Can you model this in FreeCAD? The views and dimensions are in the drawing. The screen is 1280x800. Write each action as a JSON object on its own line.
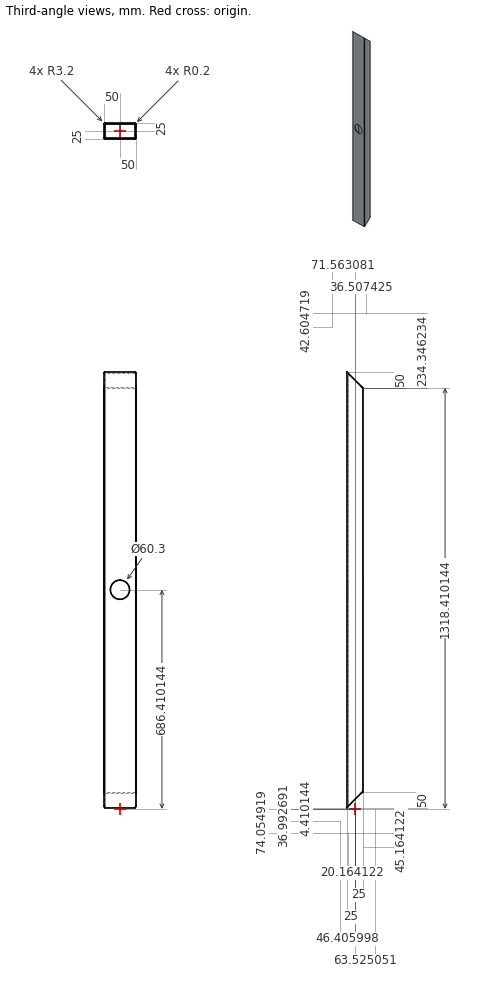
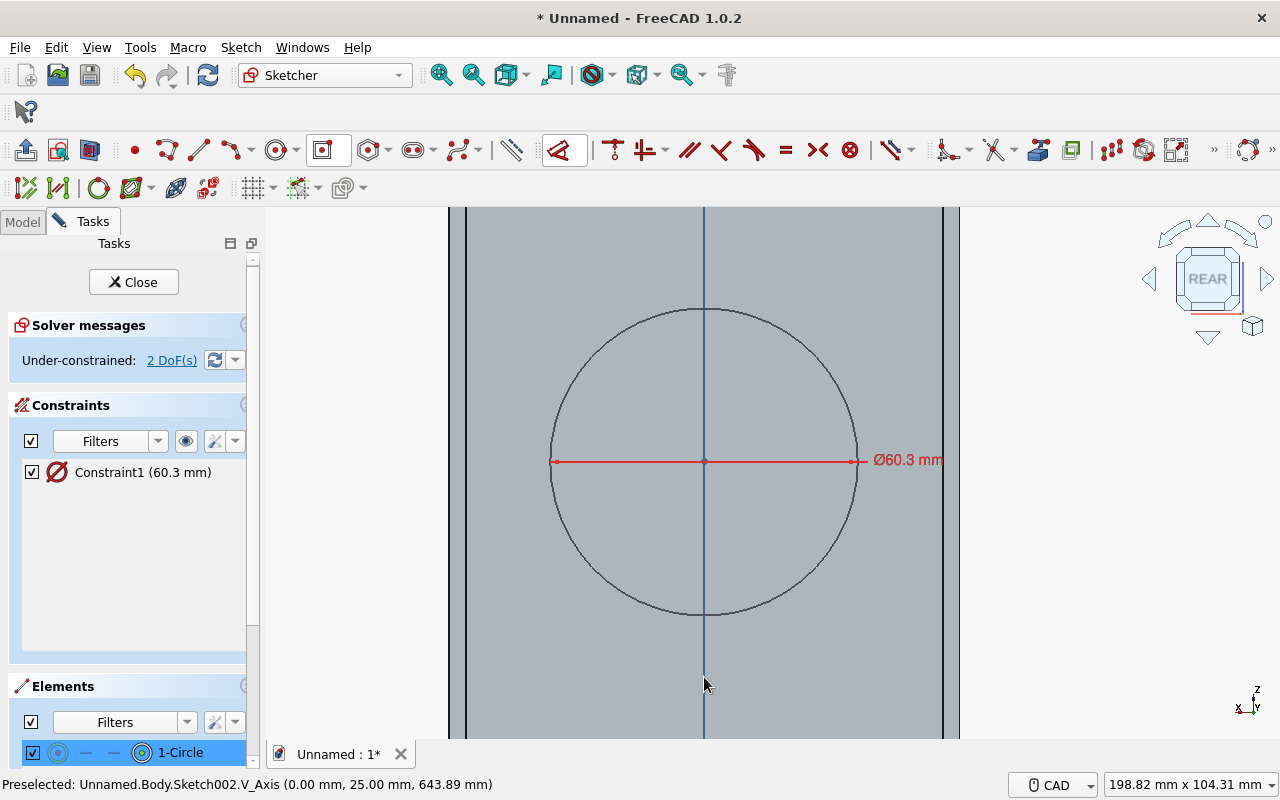
{"action": "left_click", "coordinate": [614, 150]}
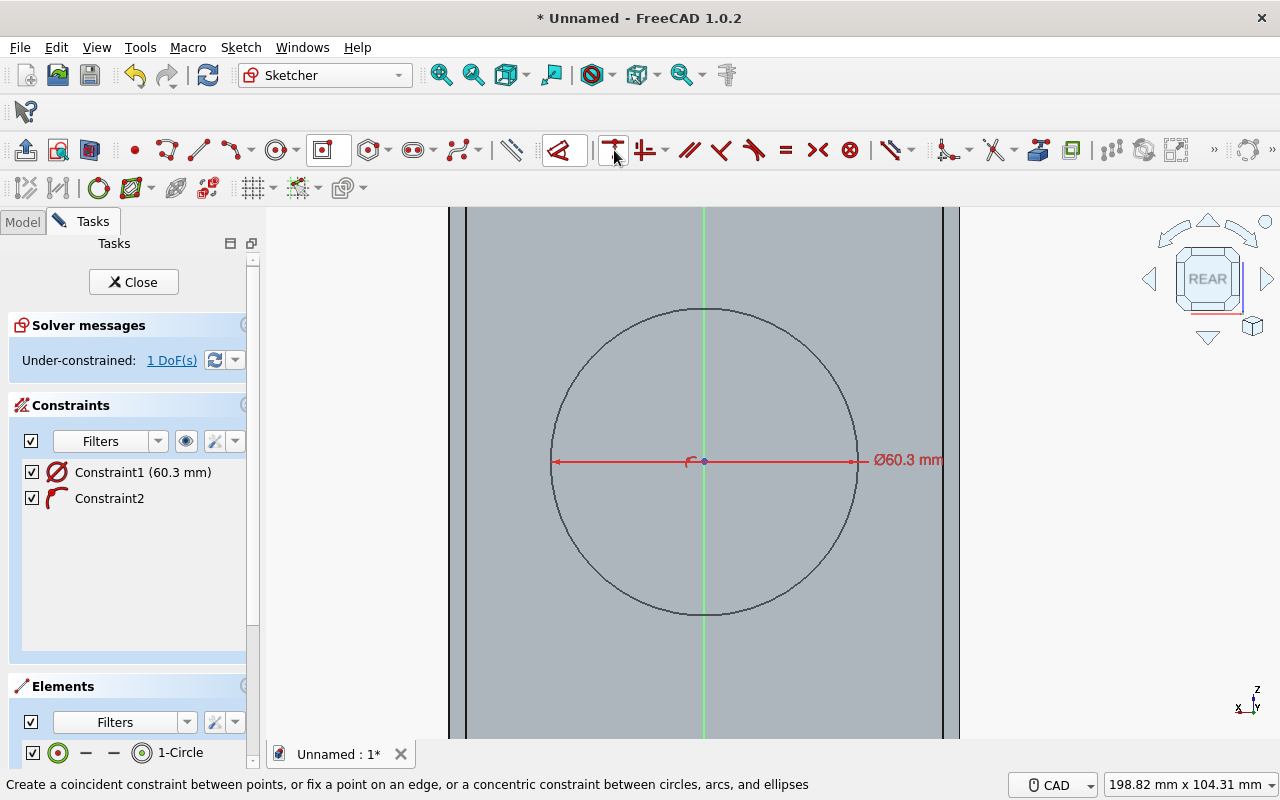
{"action": "left_click", "coordinate": [704, 462]}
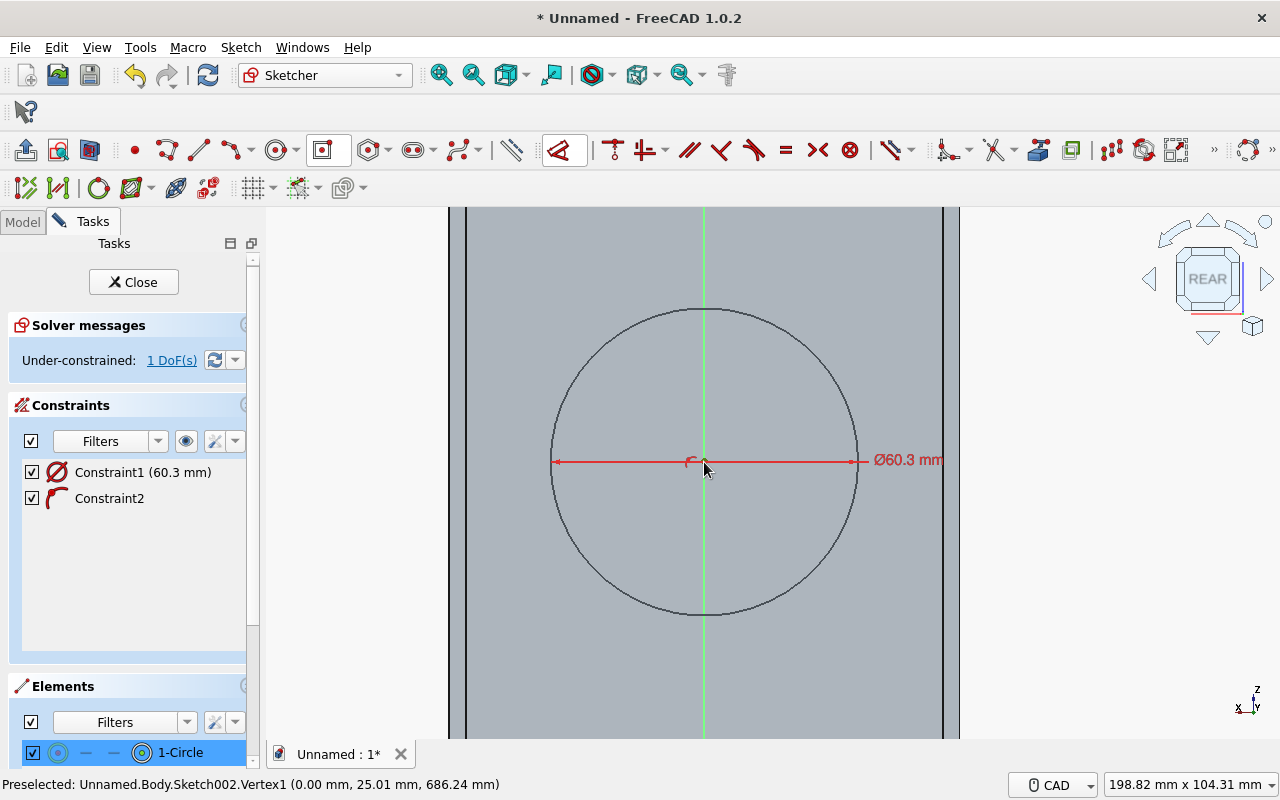
{"action": "left_click", "coordinate": [582, 150]}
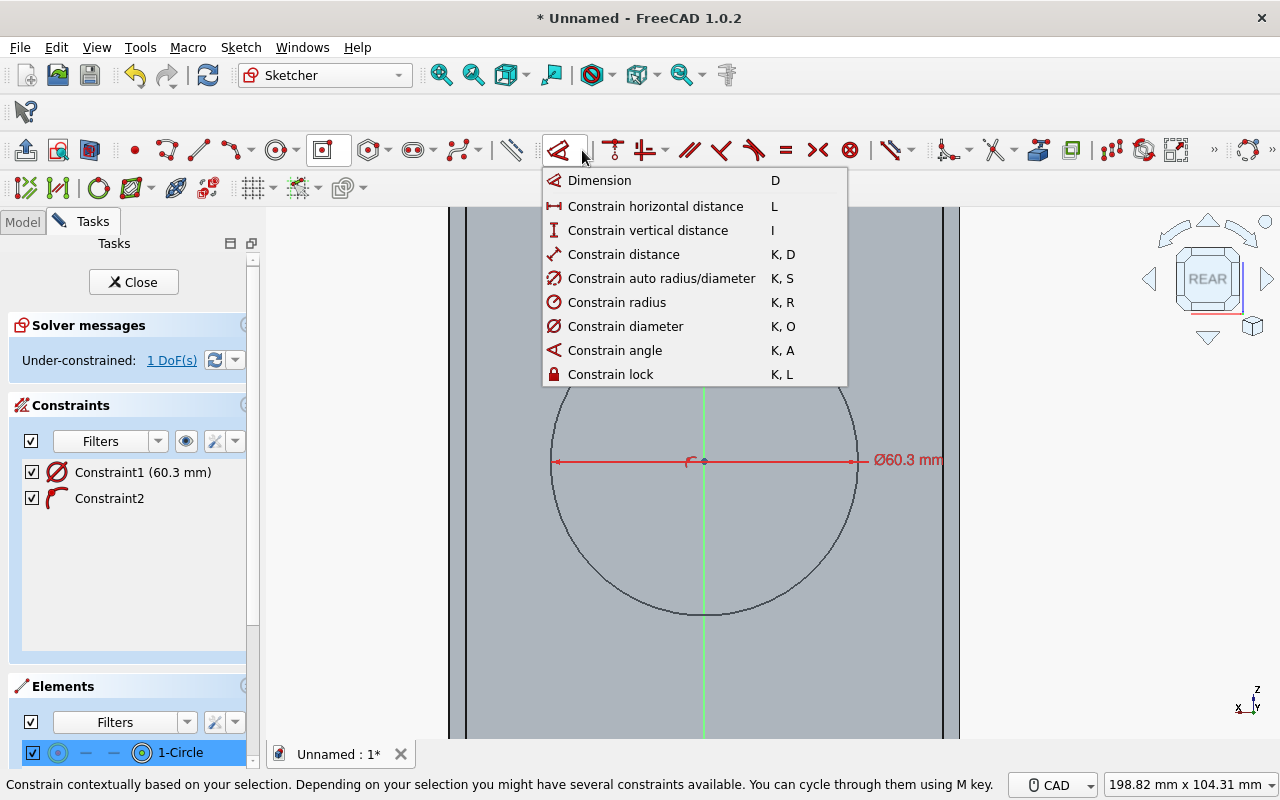
{"action": "left_click", "coordinate": [695, 230]}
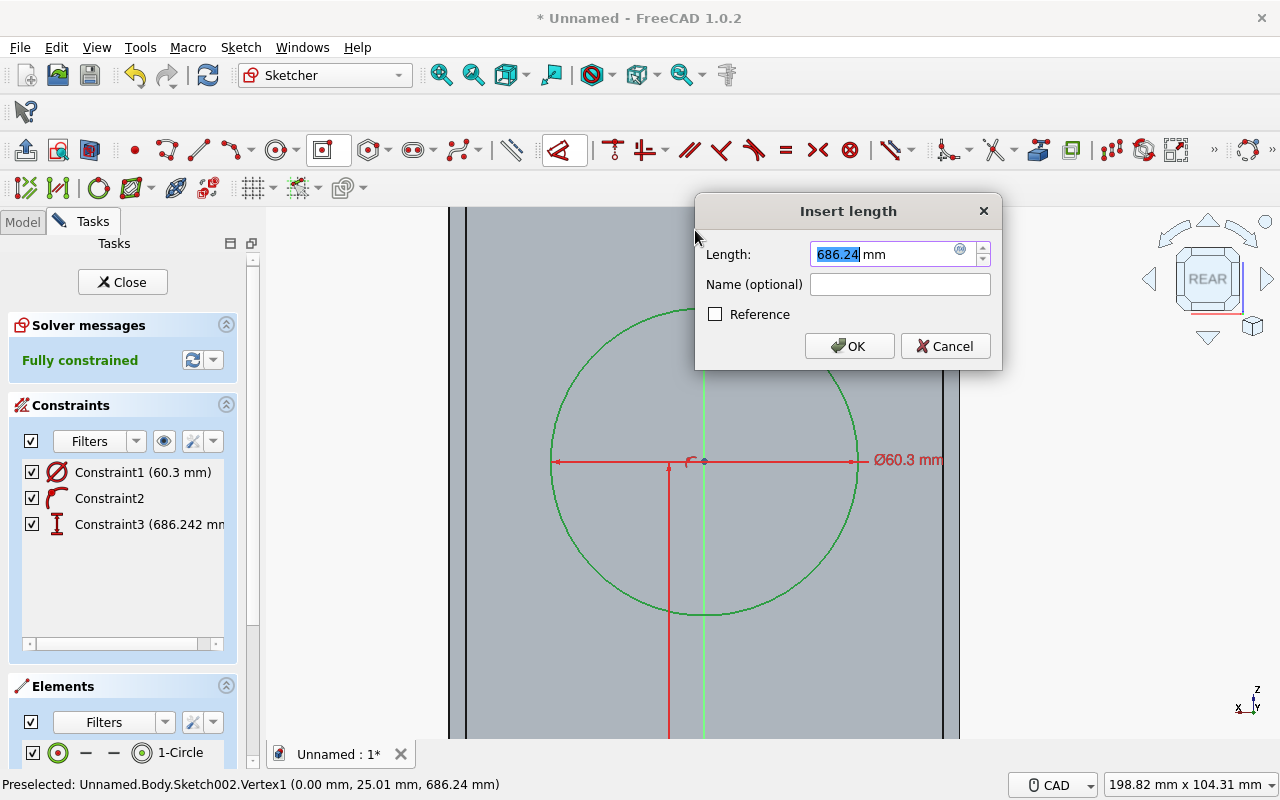
{"action": "type", "text": "686.410144"}
{"action": "key", "text": "Return"}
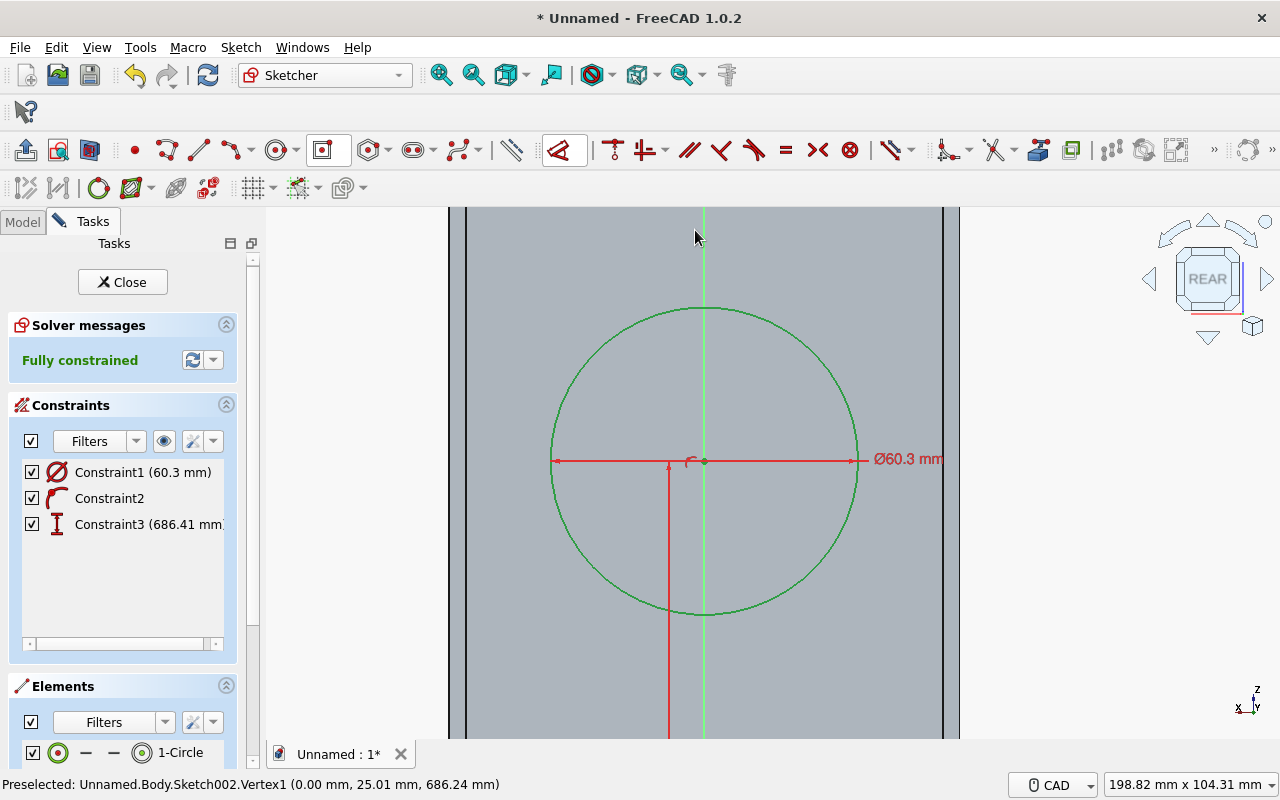
{"action": "left_click", "coordinate": [123, 282]}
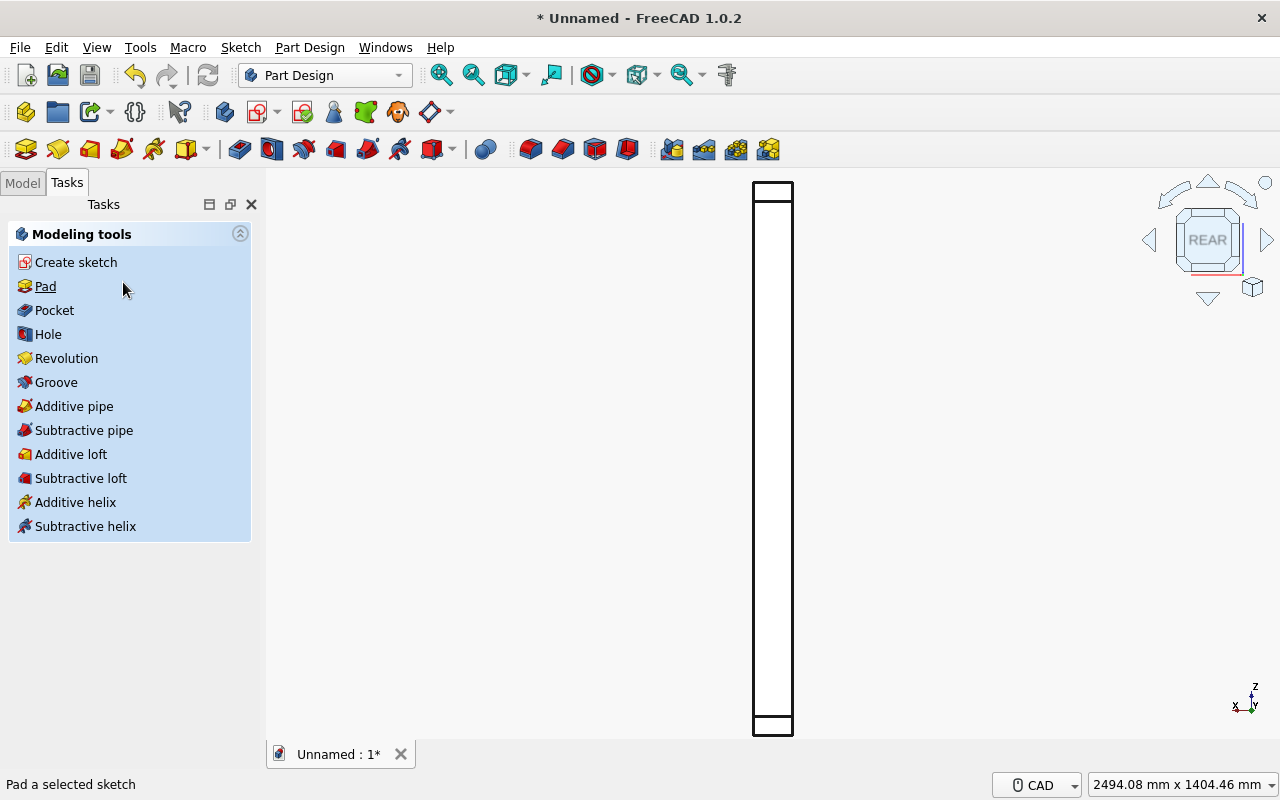
{"action": "left_click", "coordinate": [240, 150]}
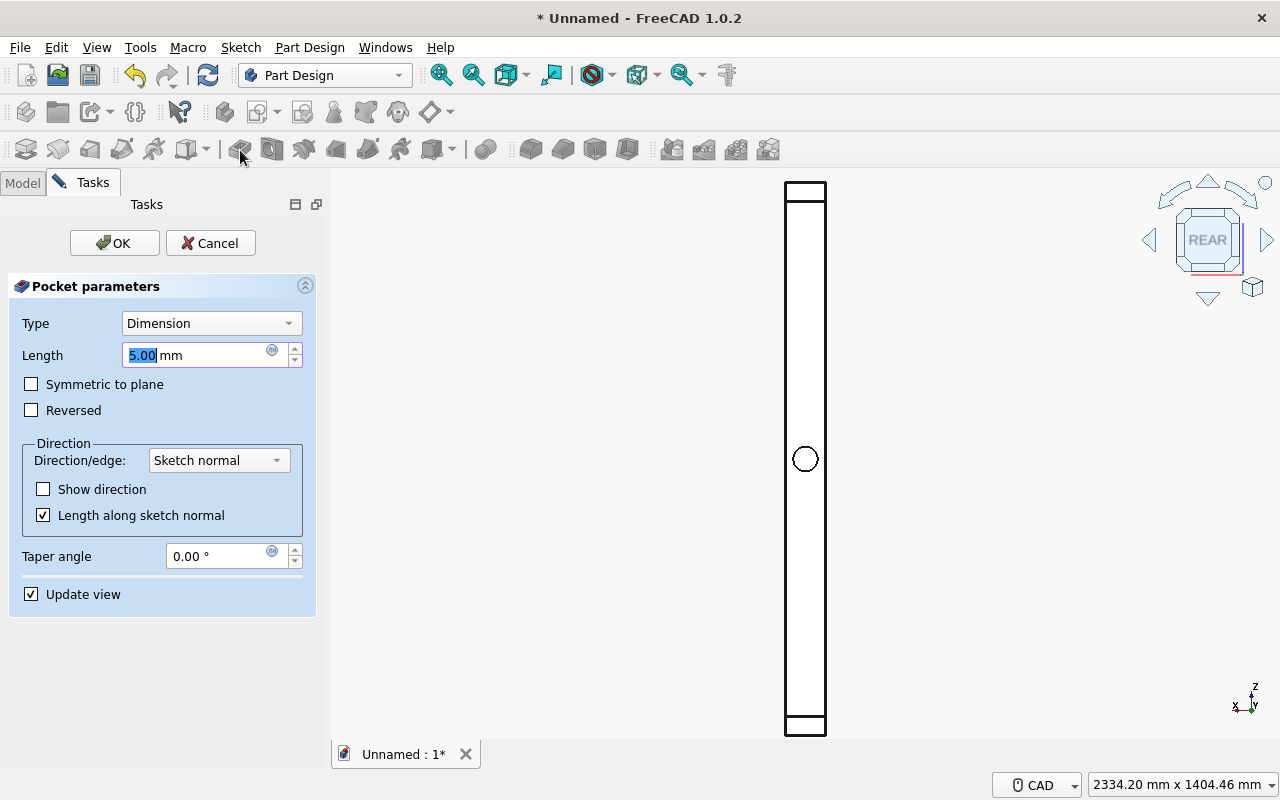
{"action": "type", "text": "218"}
{"action": "key", "text": "Tab"}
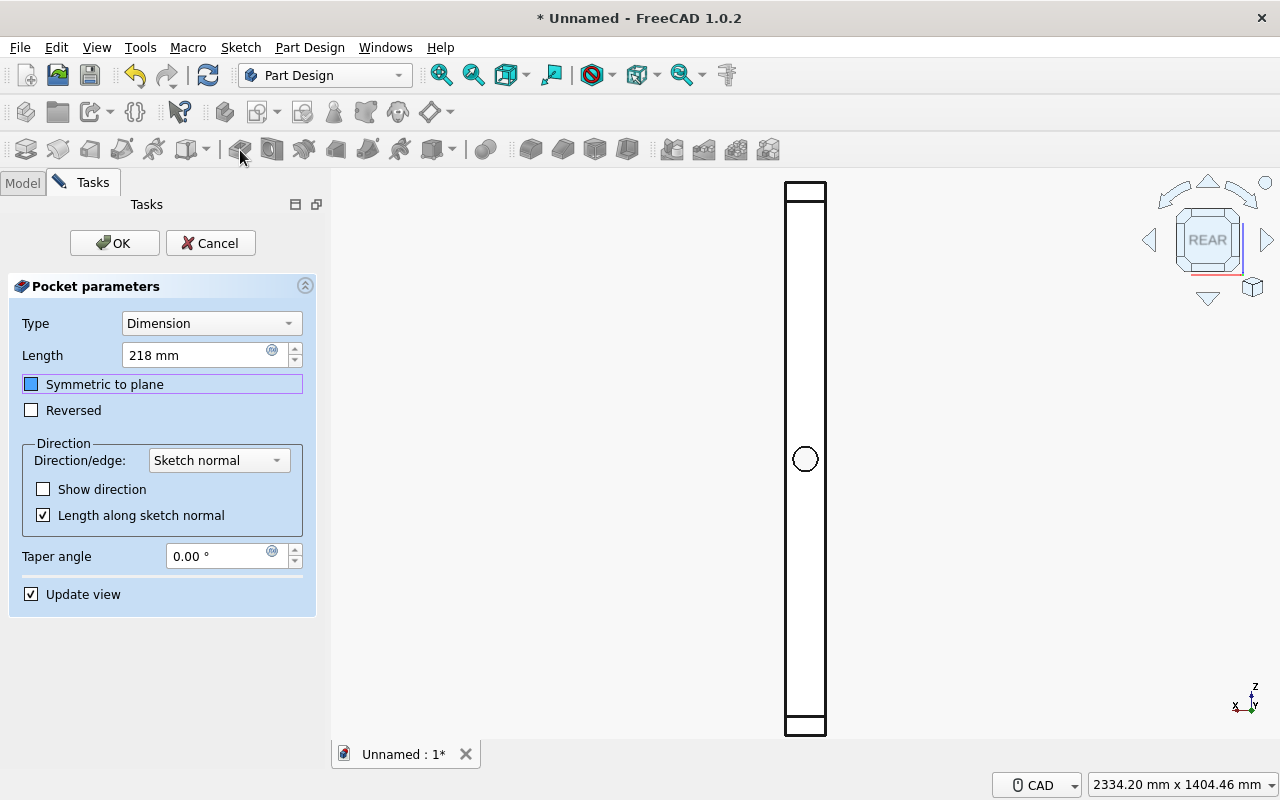
{"action": "left_click", "coordinate": [115, 243]}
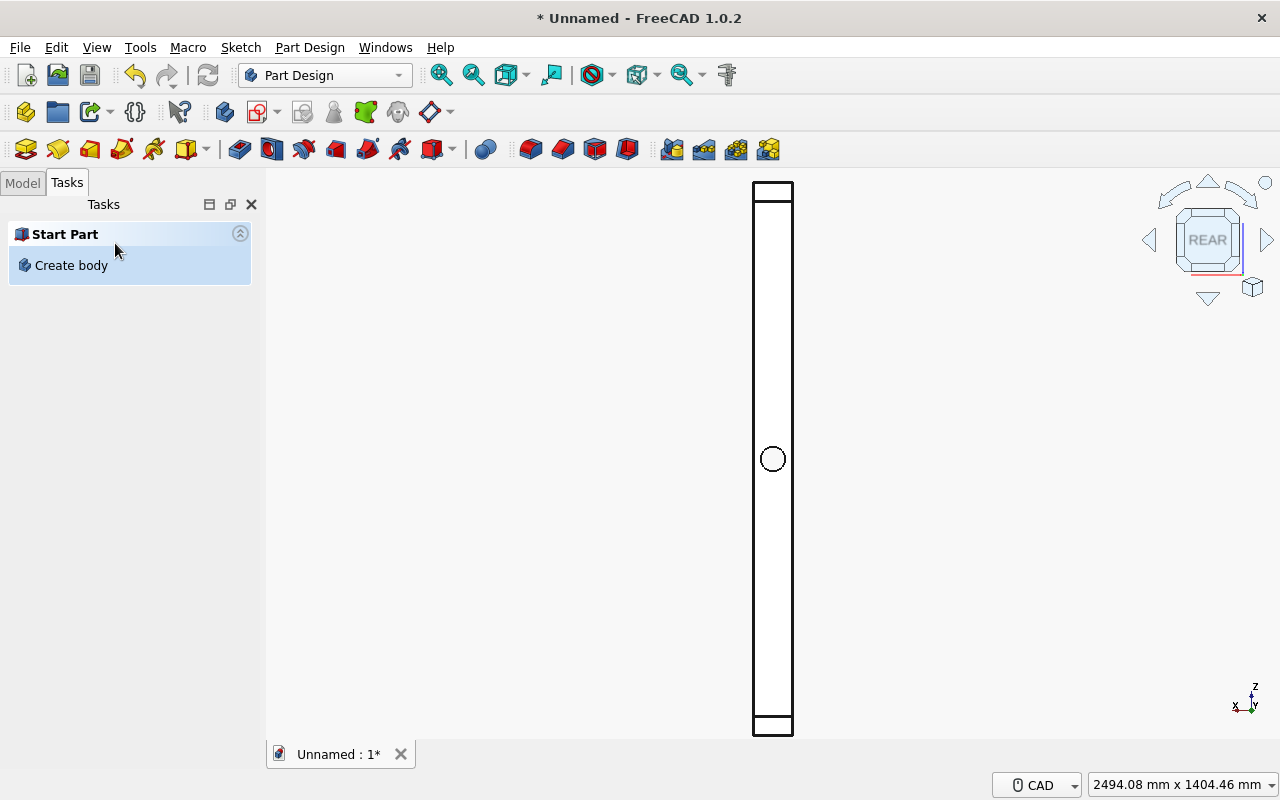
{"action": "key", "text": "0"}